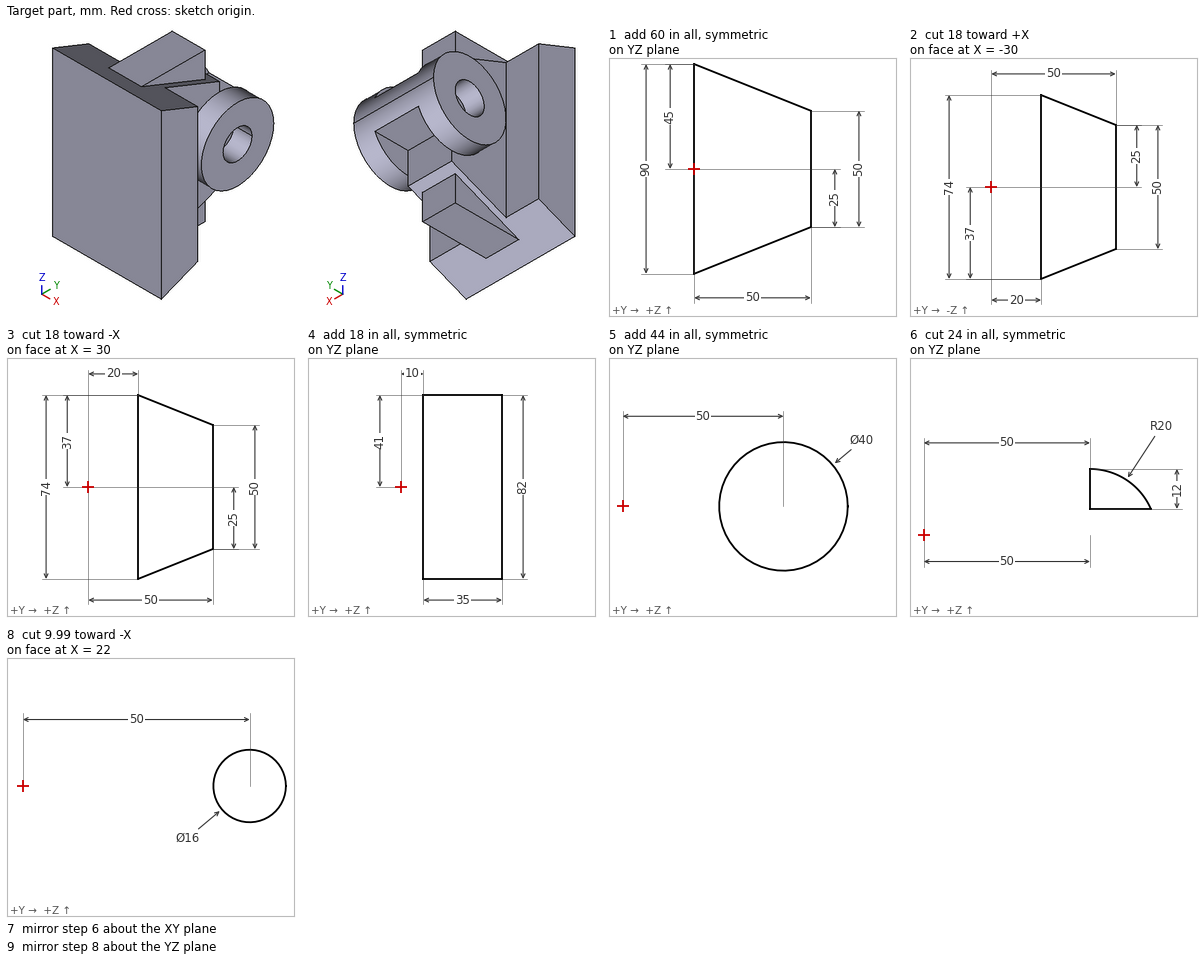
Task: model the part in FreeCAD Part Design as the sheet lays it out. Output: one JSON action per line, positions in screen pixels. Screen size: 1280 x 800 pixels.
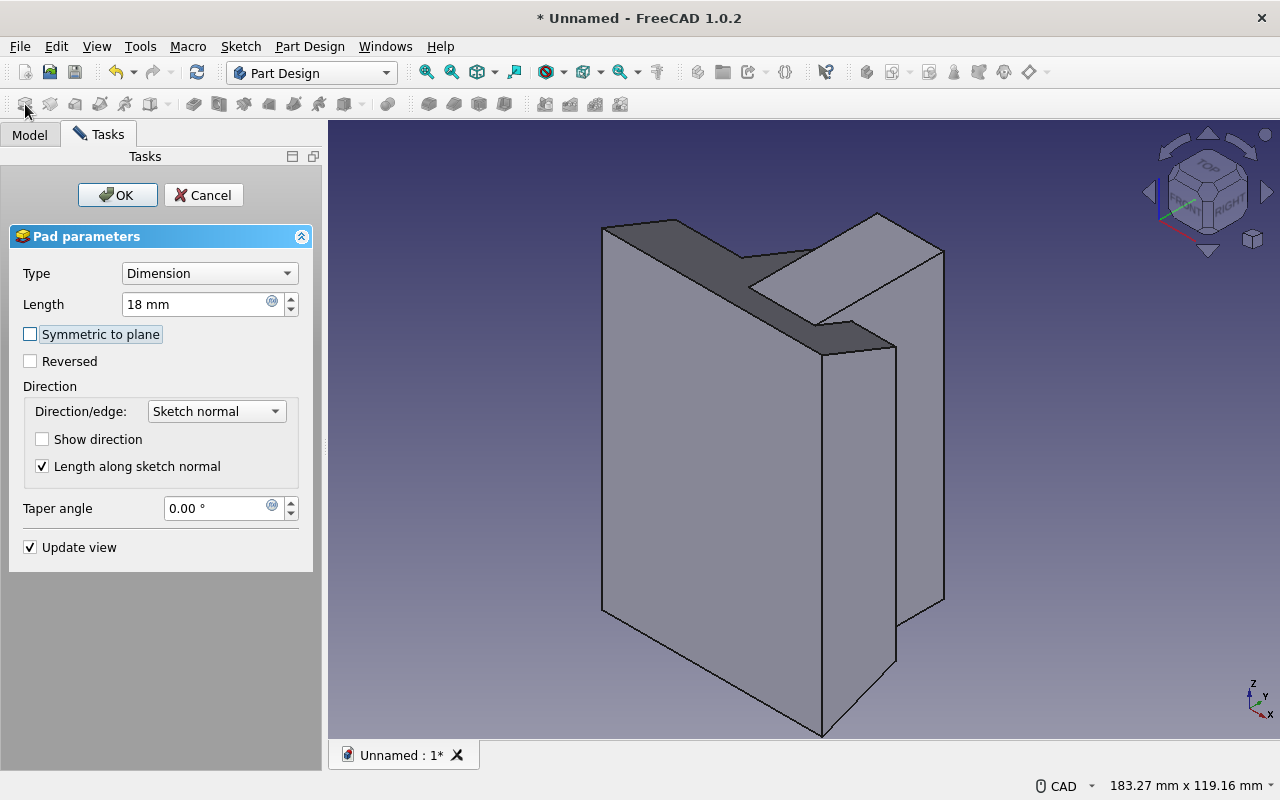
{"action": "left_click", "coordinate": [31, 334]}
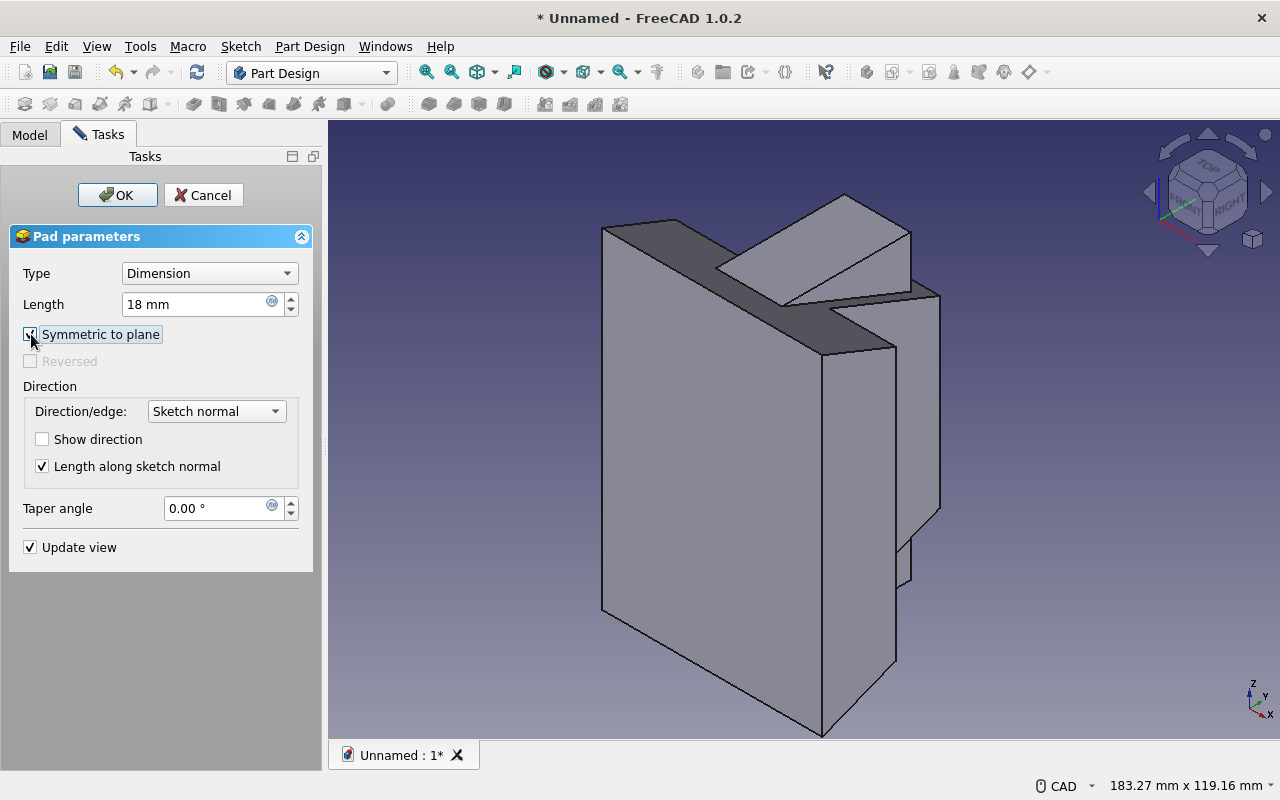
{"action": "left_click", "coordinate": [118, 195]}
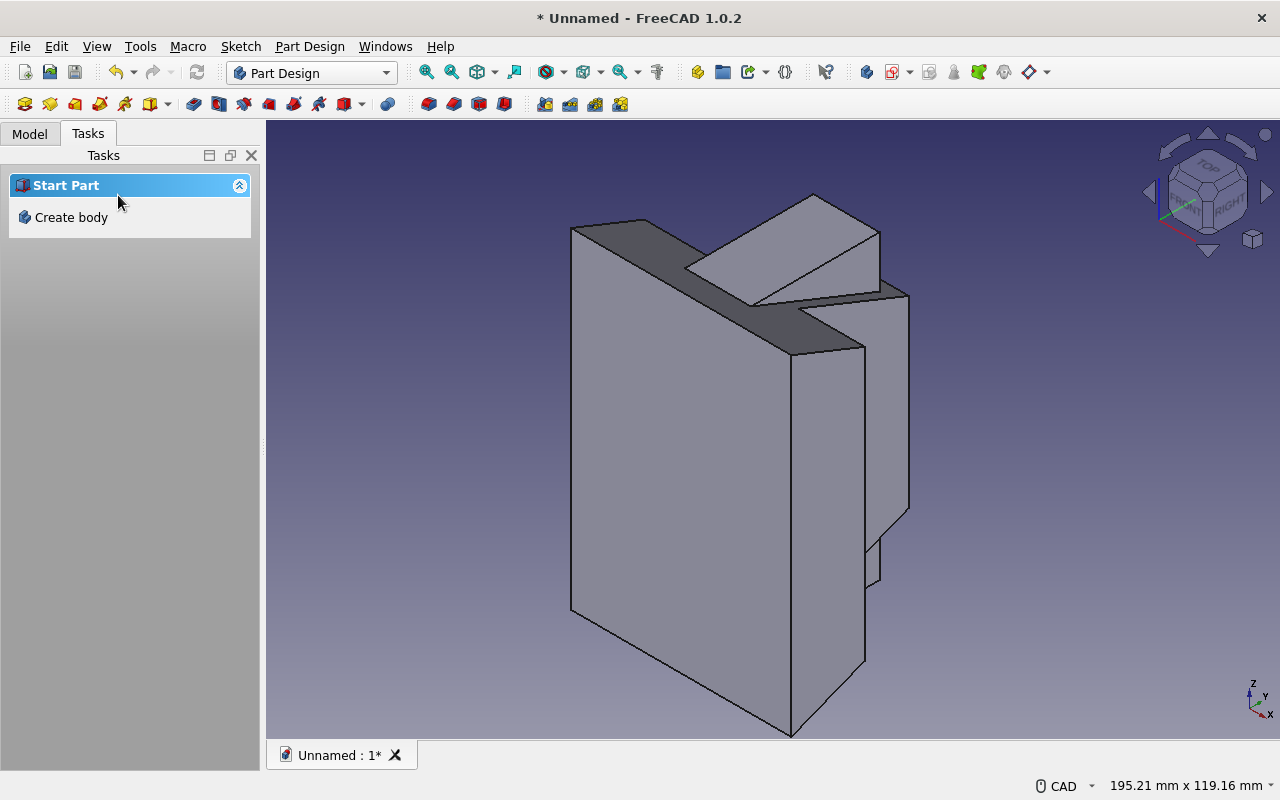
{"action": "left_click", "coordinate": [892, 72]}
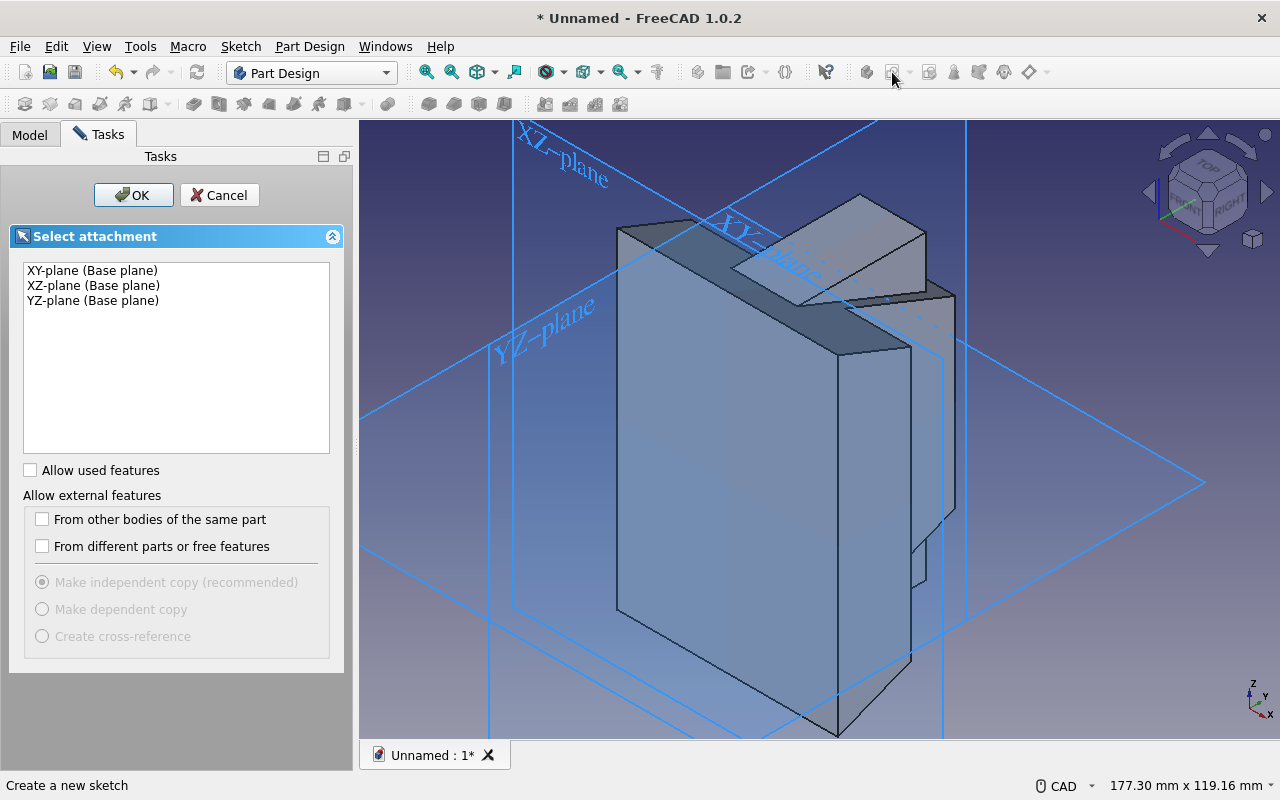
{"action": "left_click", "coordinate": [84, 300]}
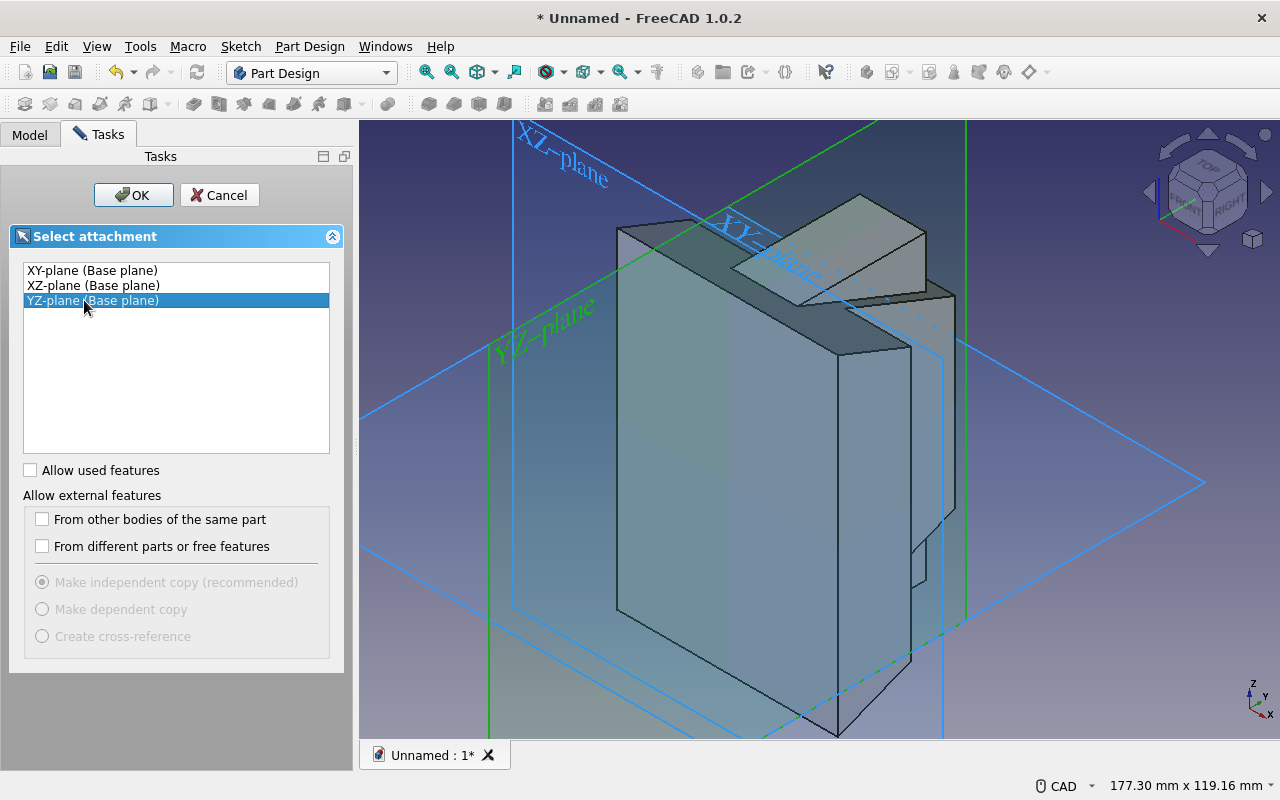
{"action": "left_click", "coordinate": [134, 195]}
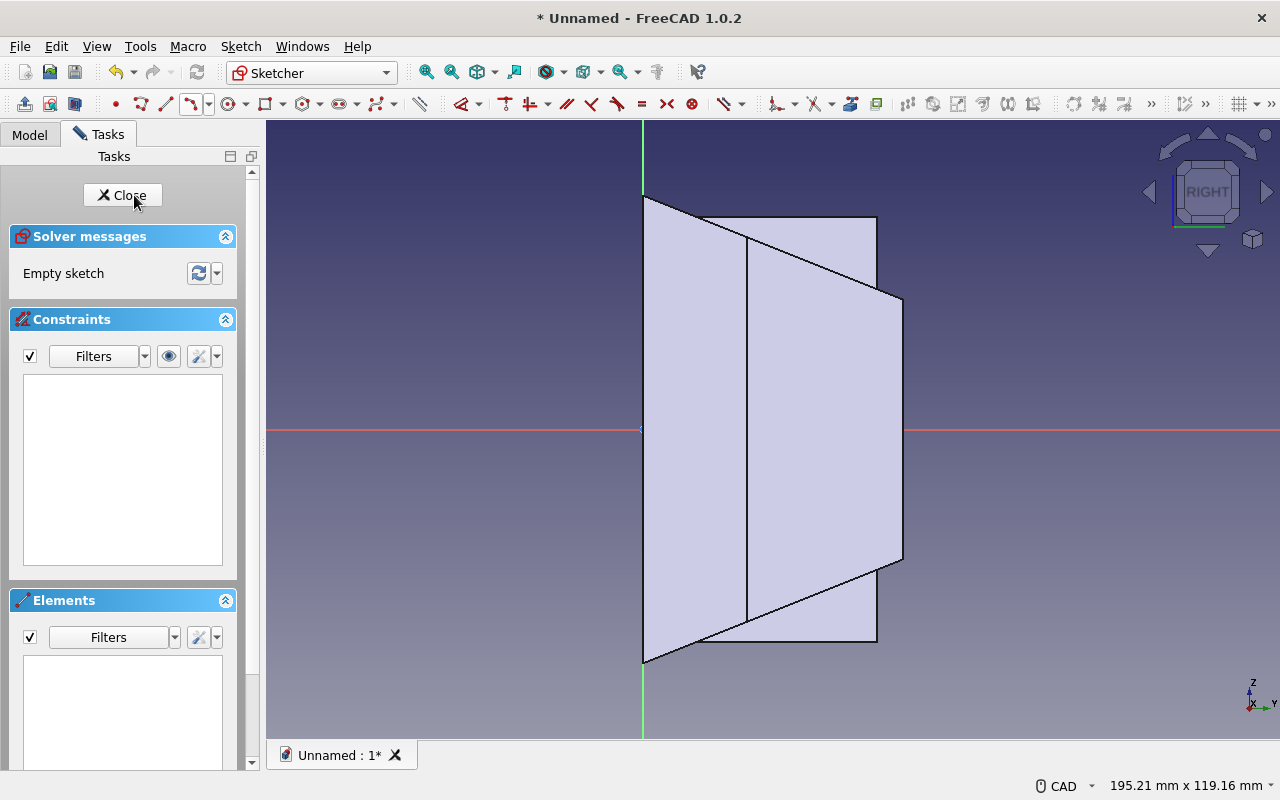
{"action": "key", "text": "q s"}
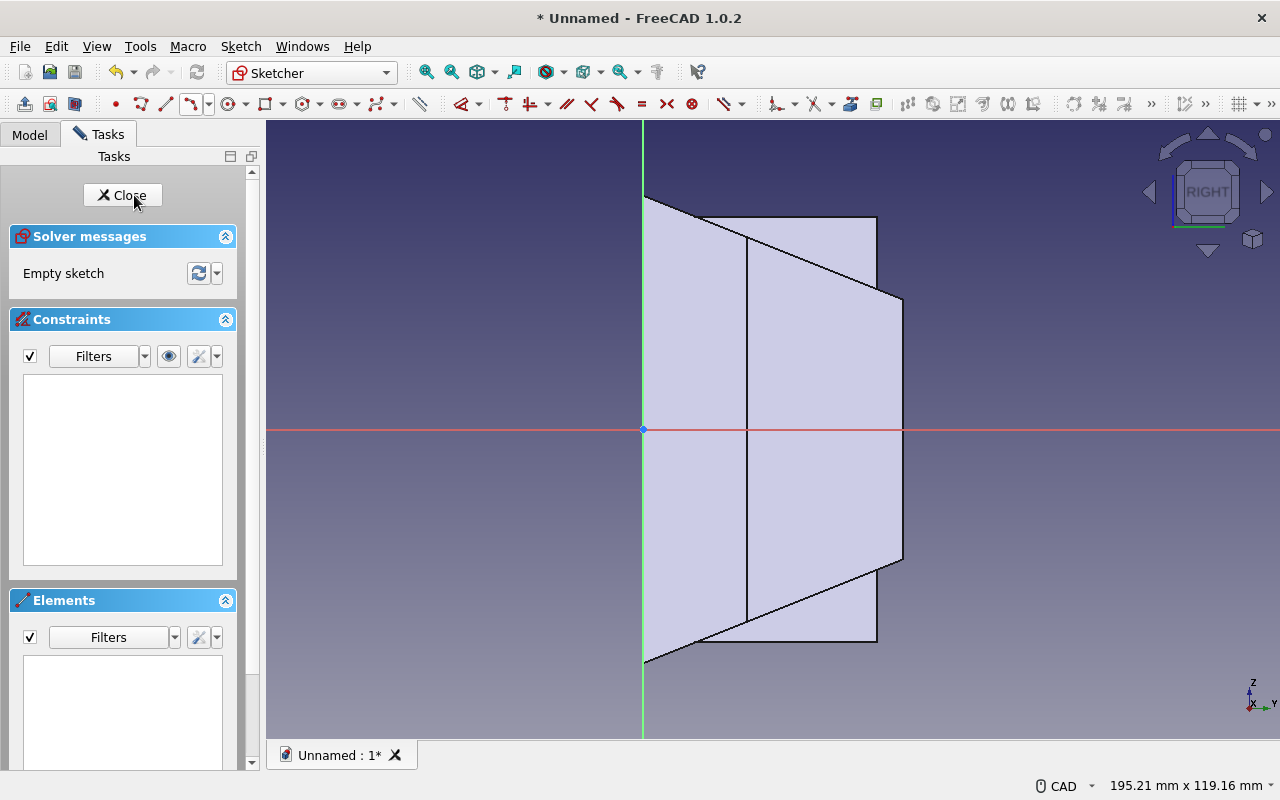
{"action": "scroll", "coordinate": [1070, 430], "scroll_direction": "up", "scroll_amount": 2}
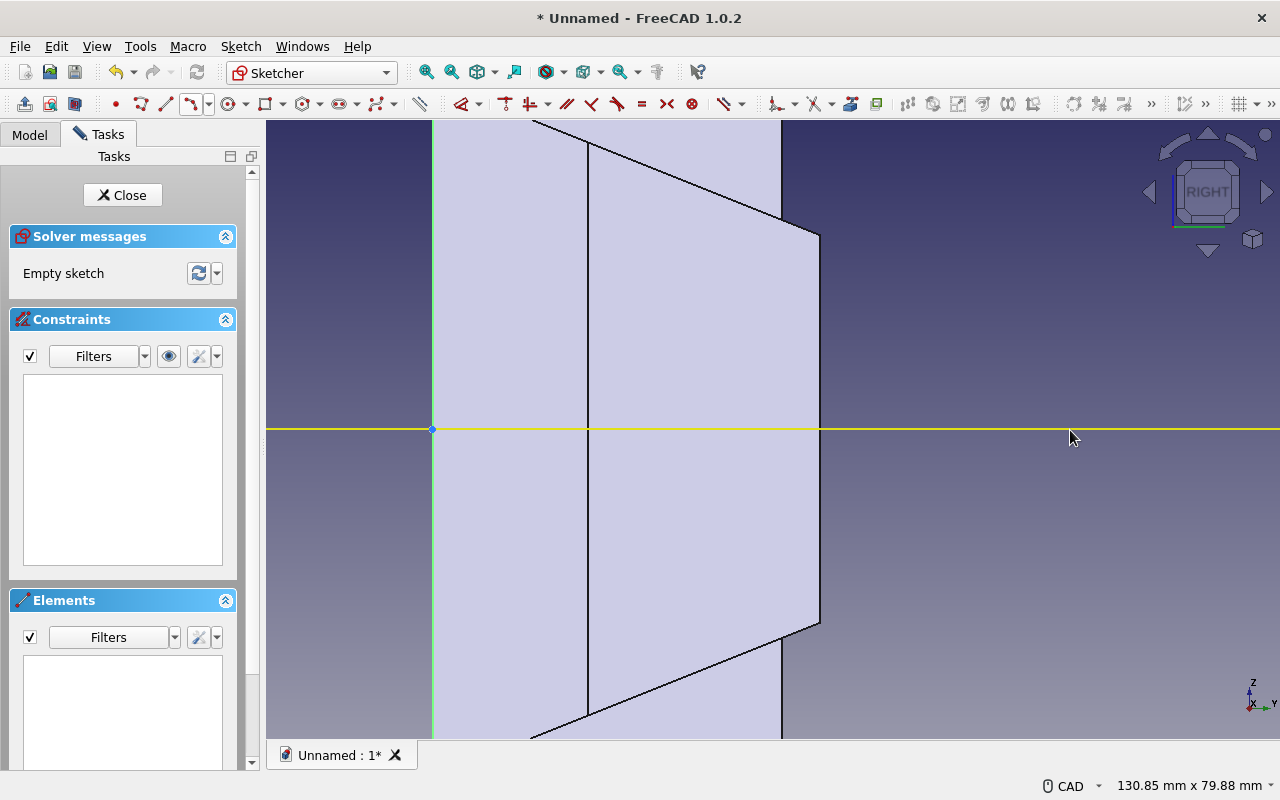
{"action": "left_click", "coordinate": [228, 104]}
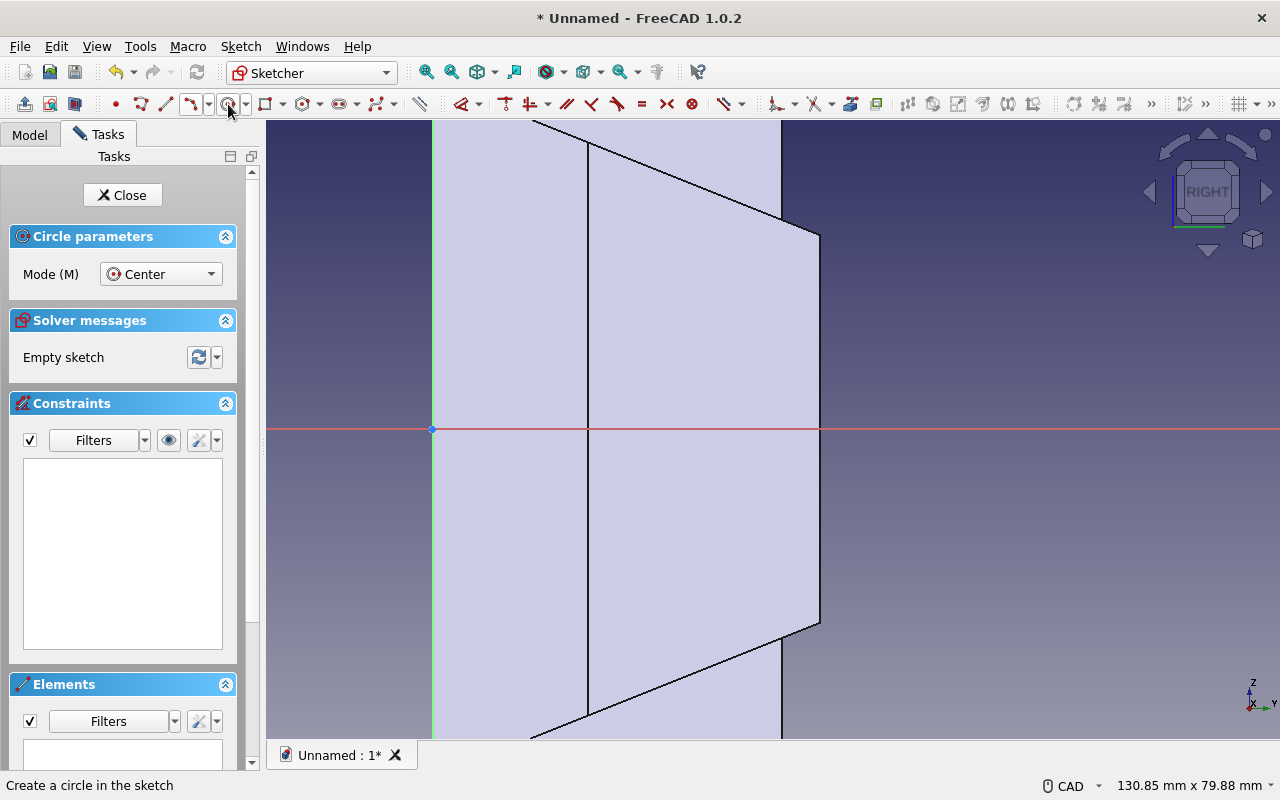
{"action": "left_click", "coordinate": [820, 429]}
{"action": "mouse_move", "coordinate": [930, 319]}